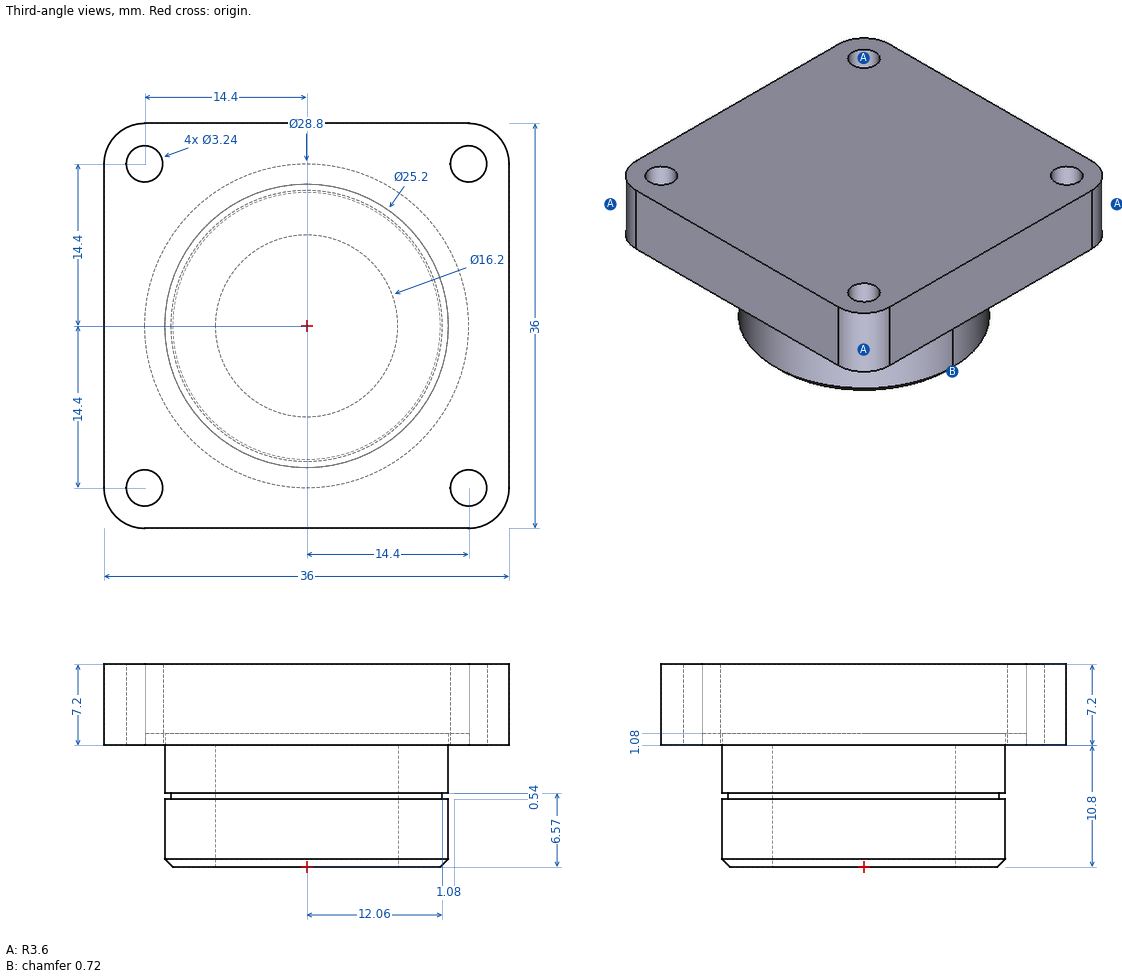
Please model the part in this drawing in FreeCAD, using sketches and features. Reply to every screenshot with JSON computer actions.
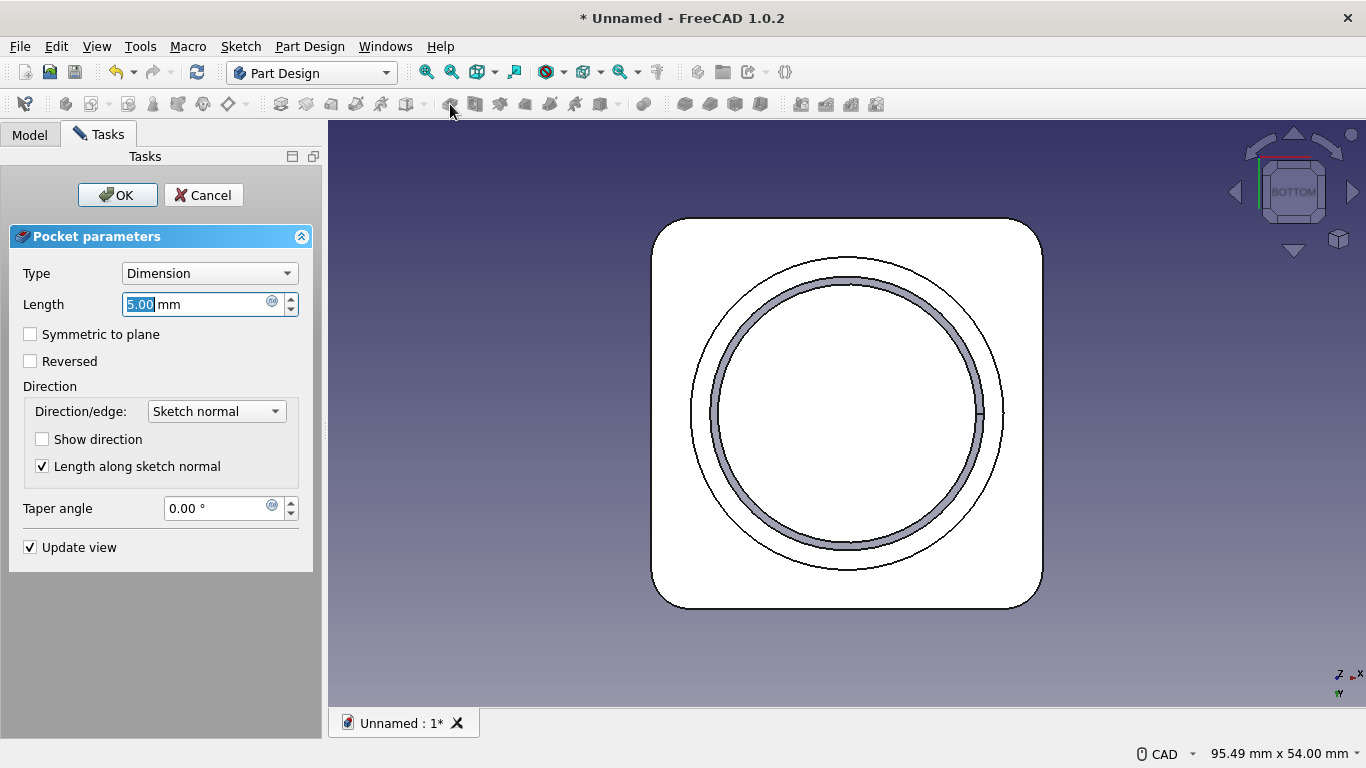
{"action": "type", "text": "1.08"}
{"action": "key", "text": "Tab"}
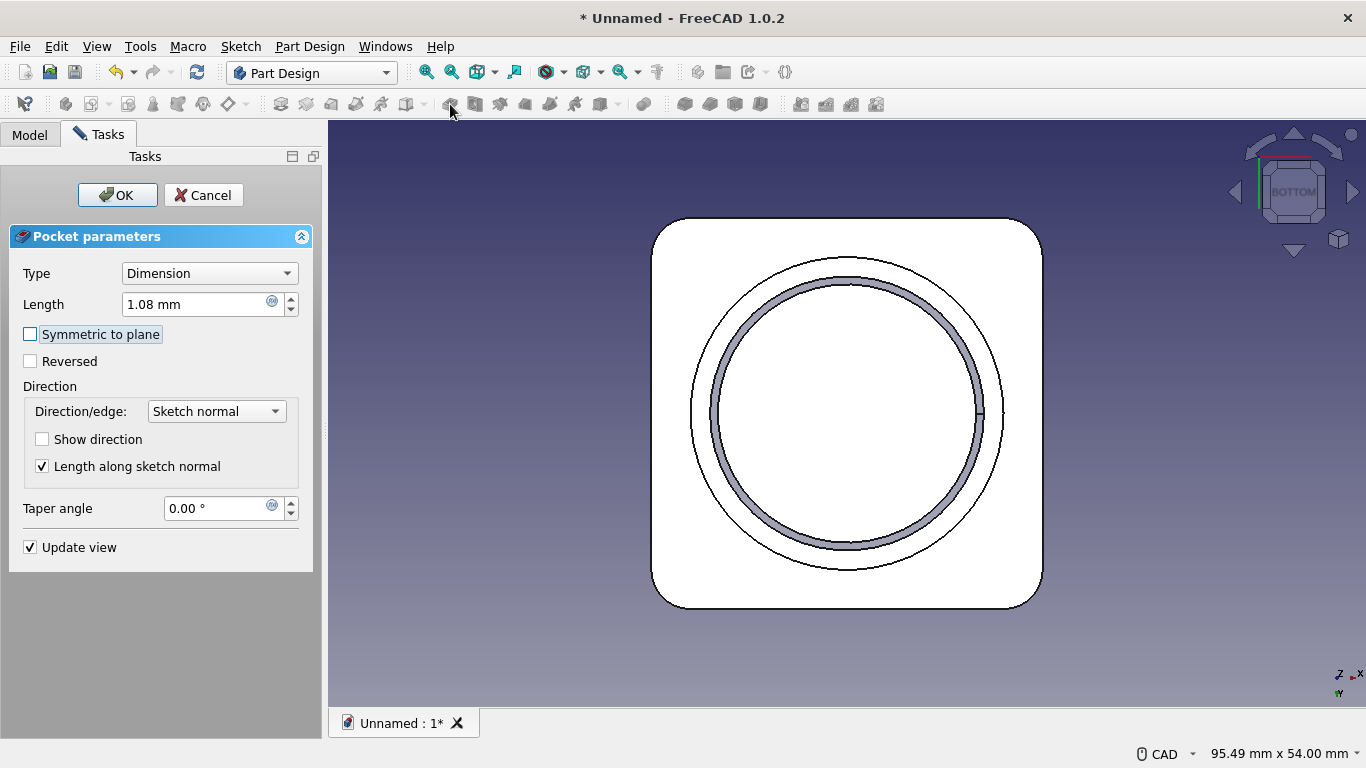
{"action": "left_click", "coordinate": [118, 195]}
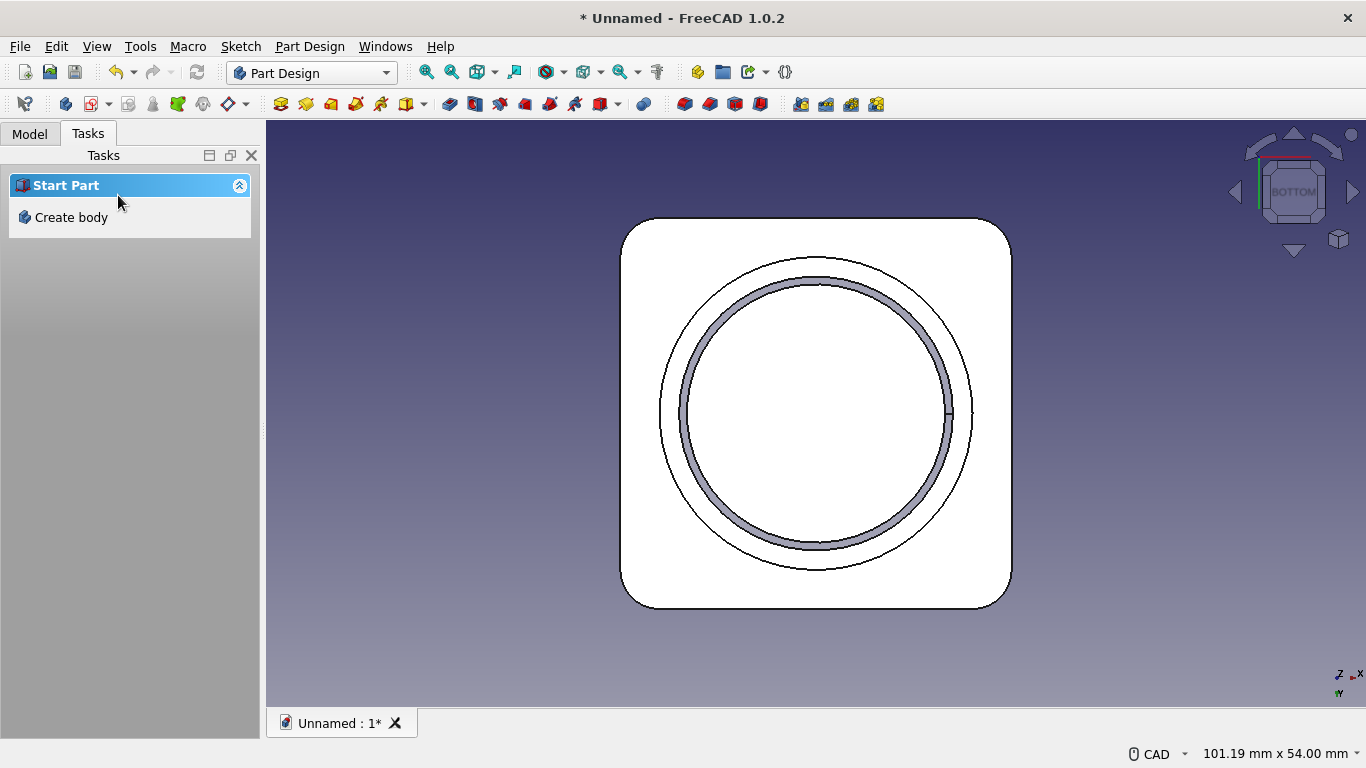
{"action": "left_click", "coordinate": [90, 104]}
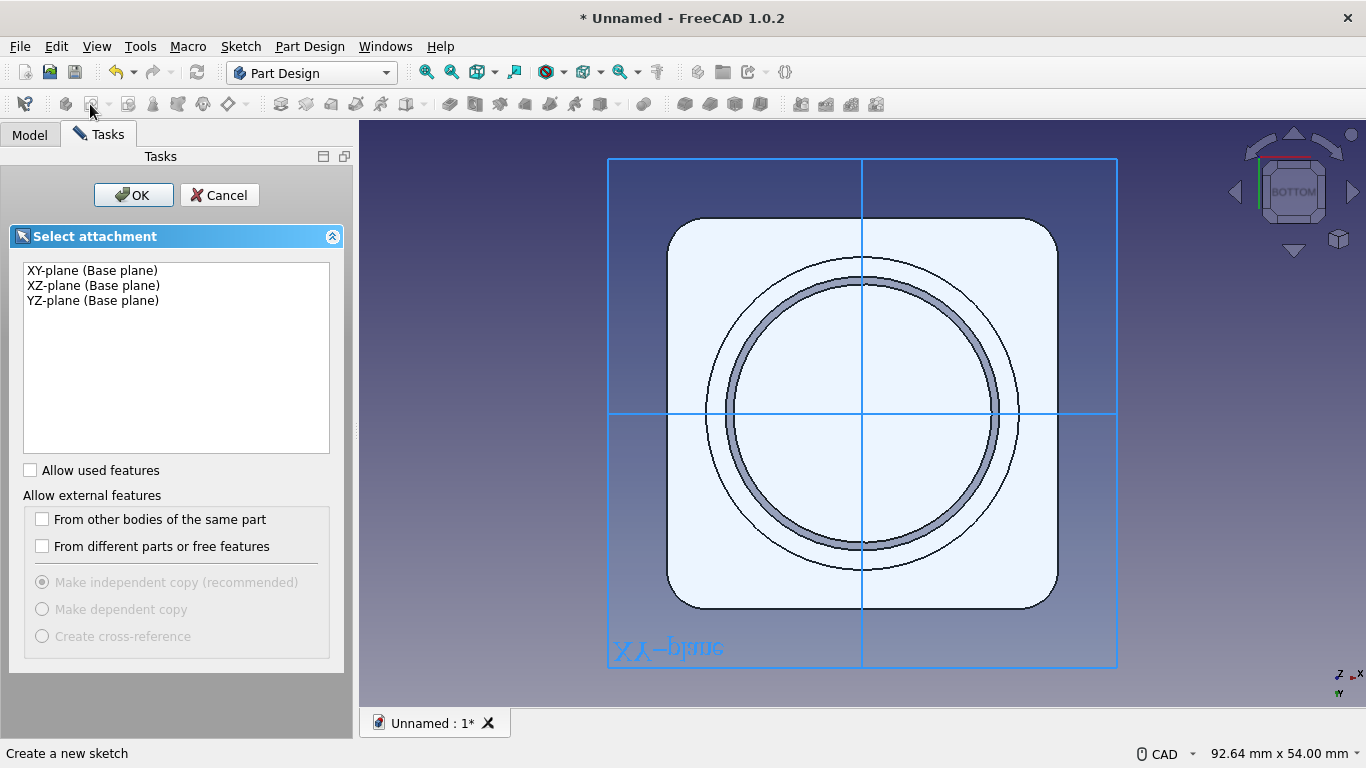
{"action": "left_click", "coordinate": [84, 286]}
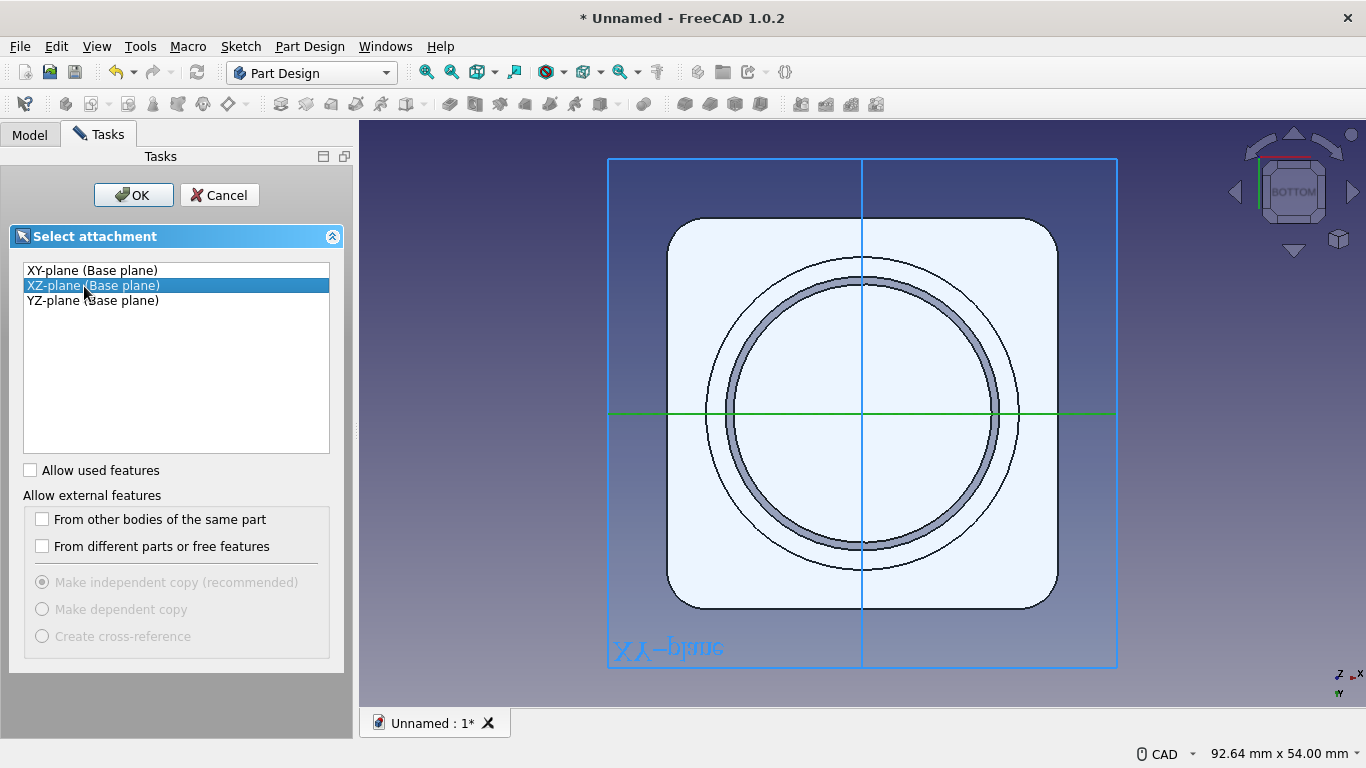
{"action": "left_click", "coordinate": [134, 195]}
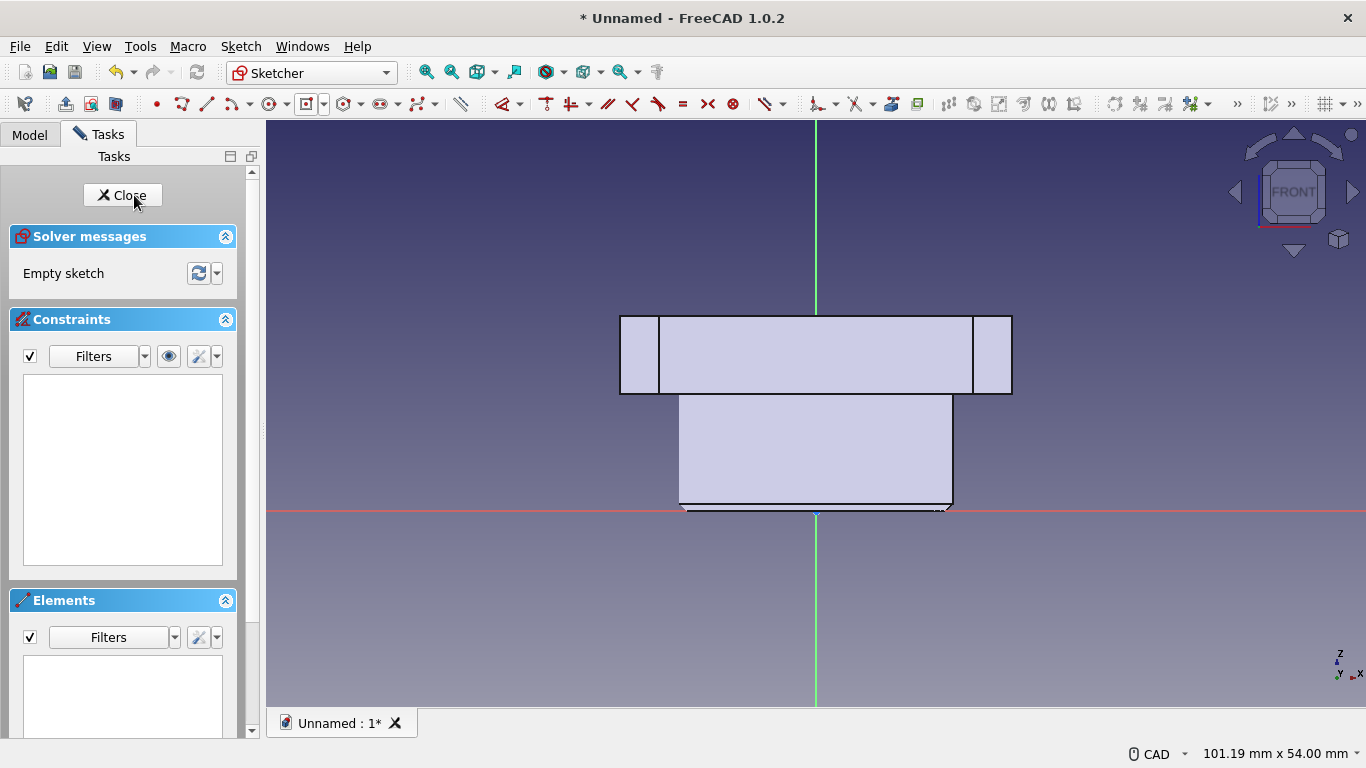
{"action": "key", "text": "q s"}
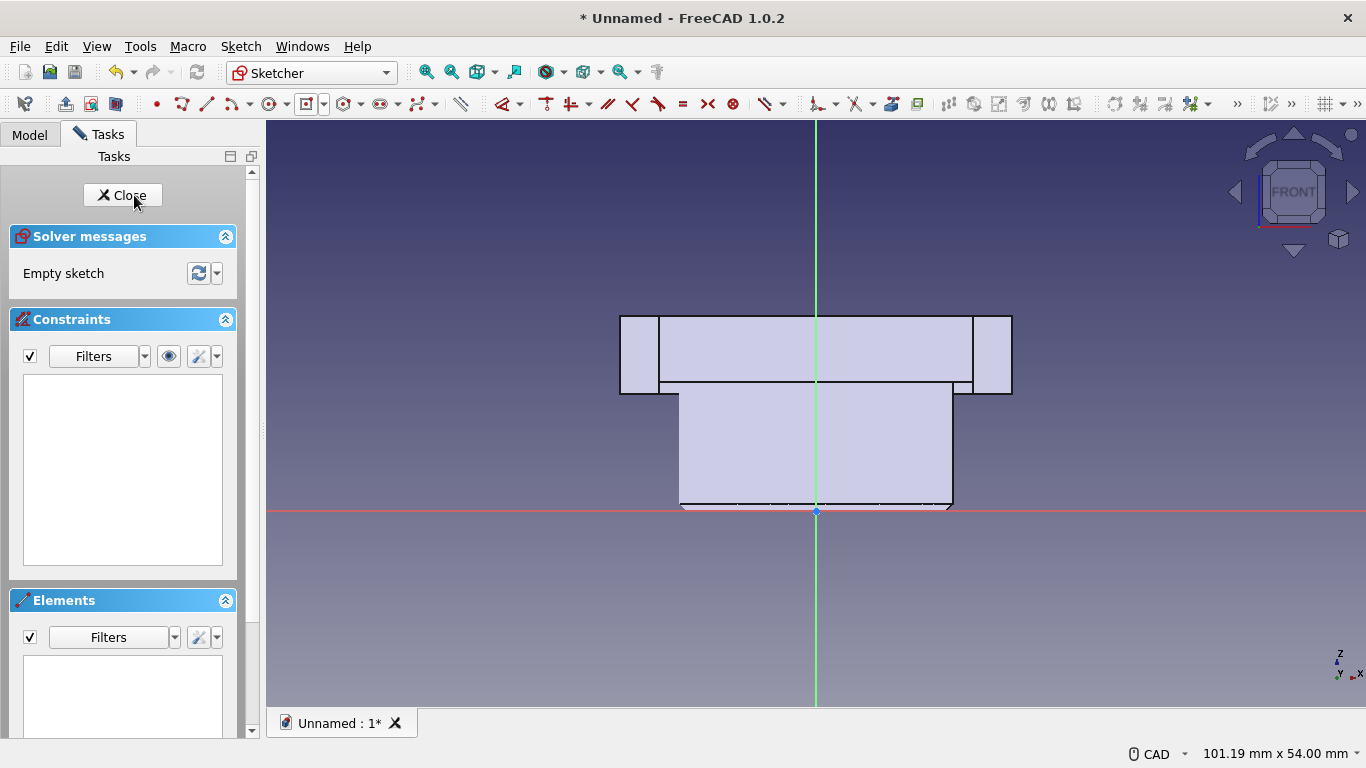
{"action": "scroll", "coordinate": [964, 444], "scroll_direction": "up", "scroll_amount": 15}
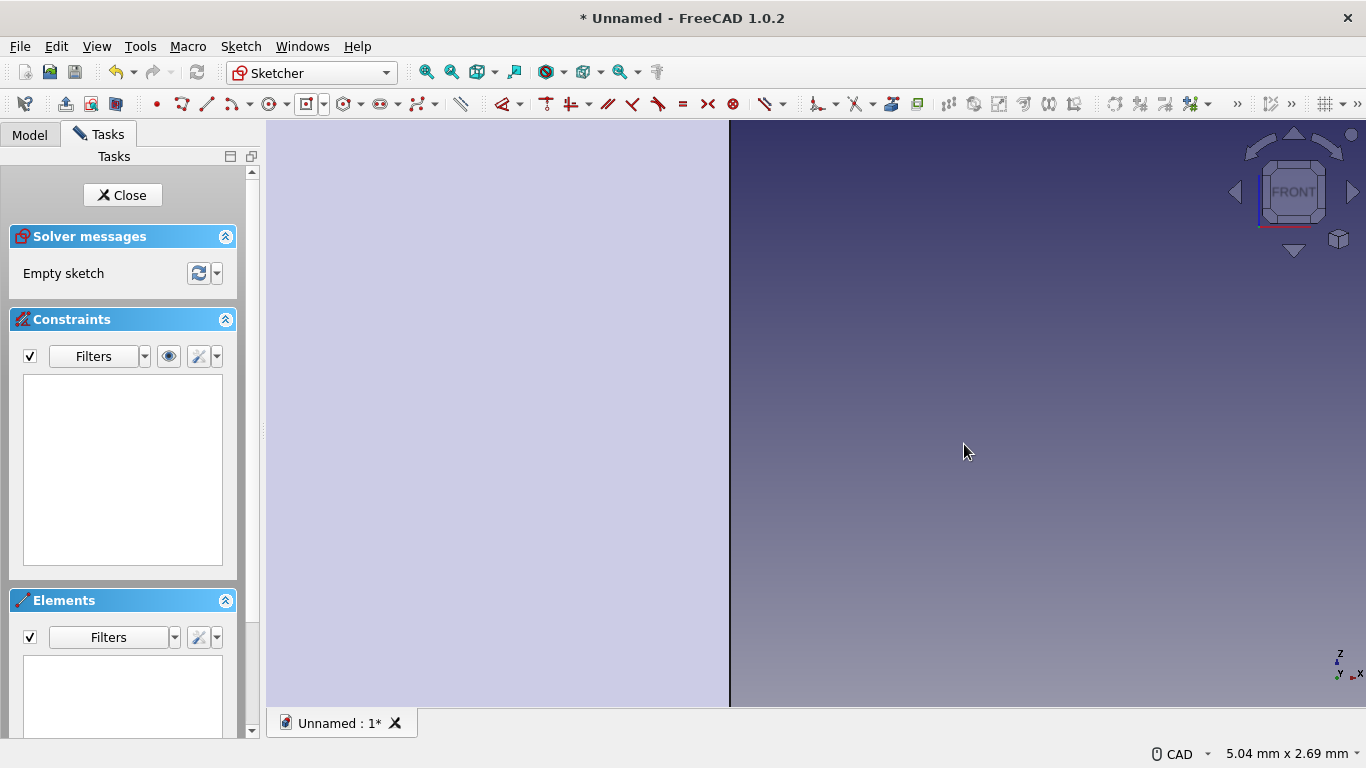
{"action": "scroll", "coordinate": [720, 409], "scroll_direction": "up", "scroll_amount": 5}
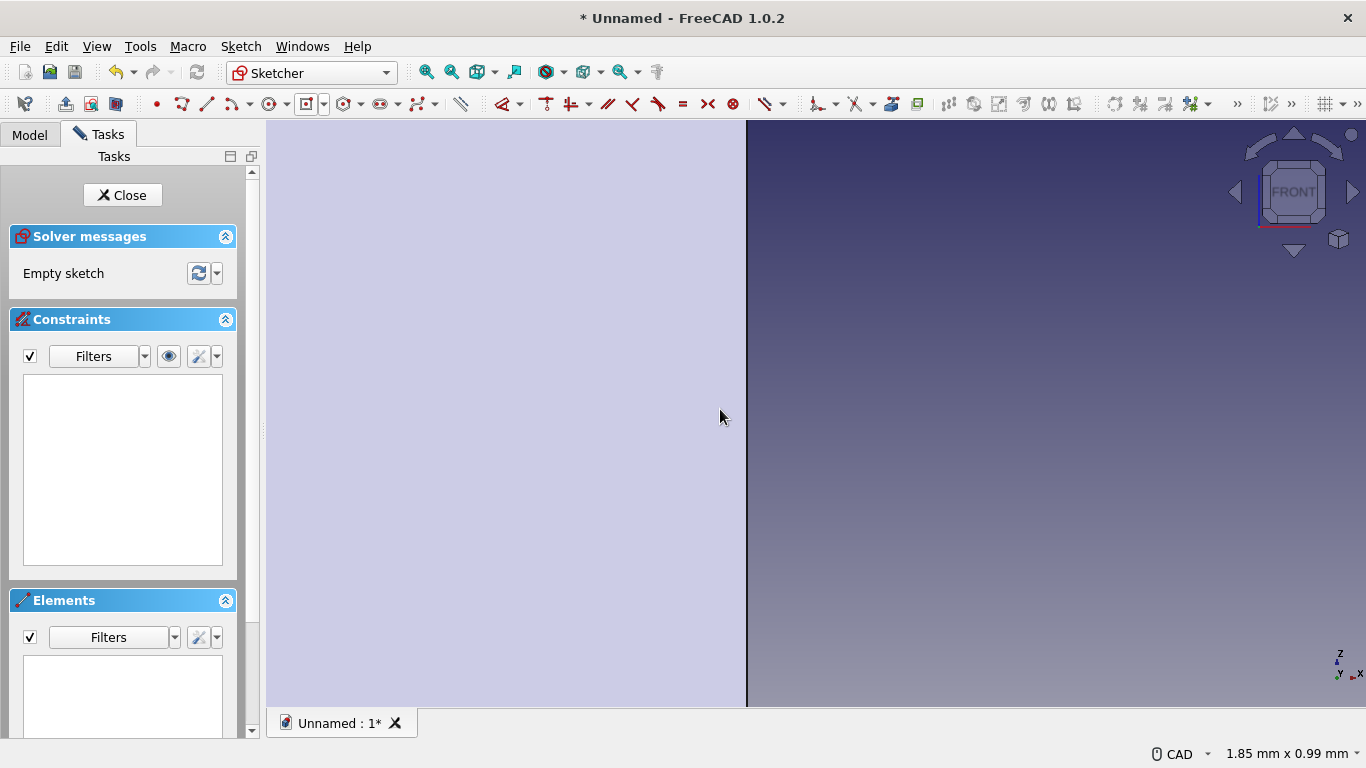
{"action": "left_click", "coordinate": [324, 104]}